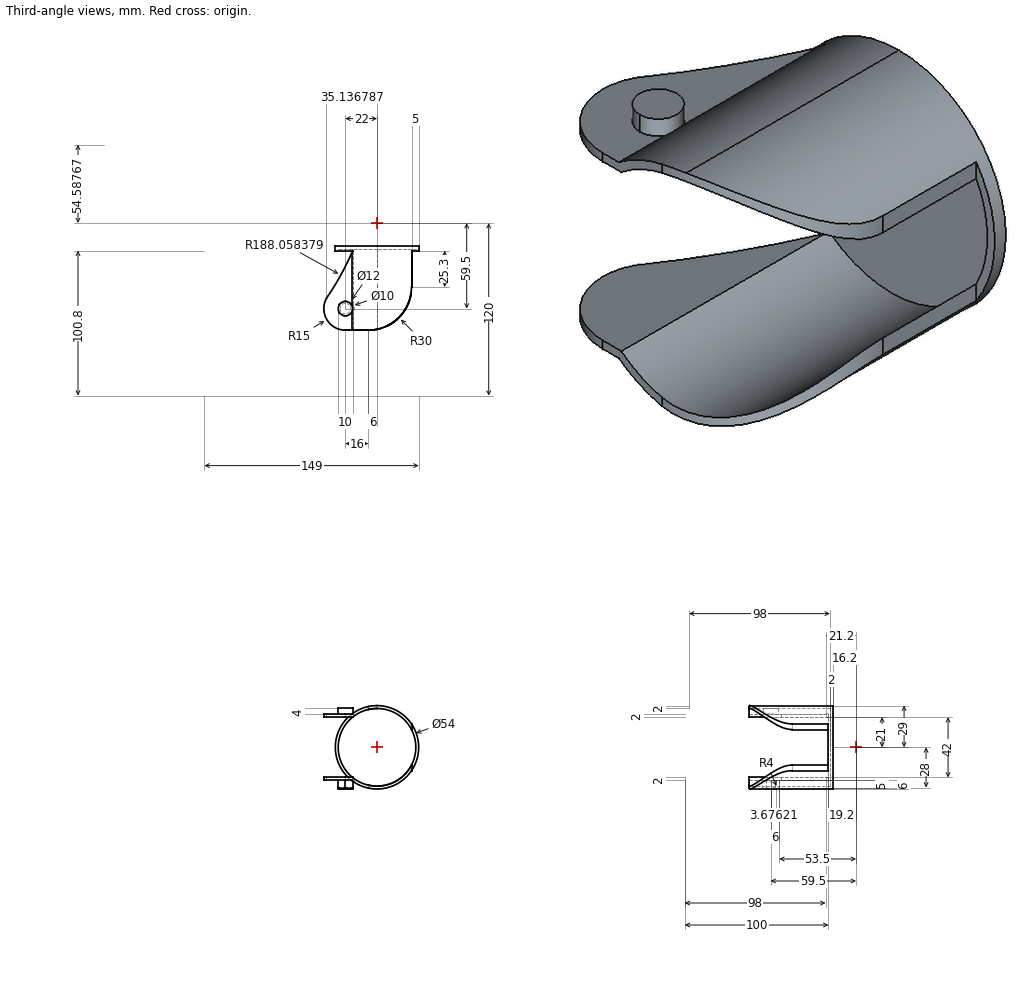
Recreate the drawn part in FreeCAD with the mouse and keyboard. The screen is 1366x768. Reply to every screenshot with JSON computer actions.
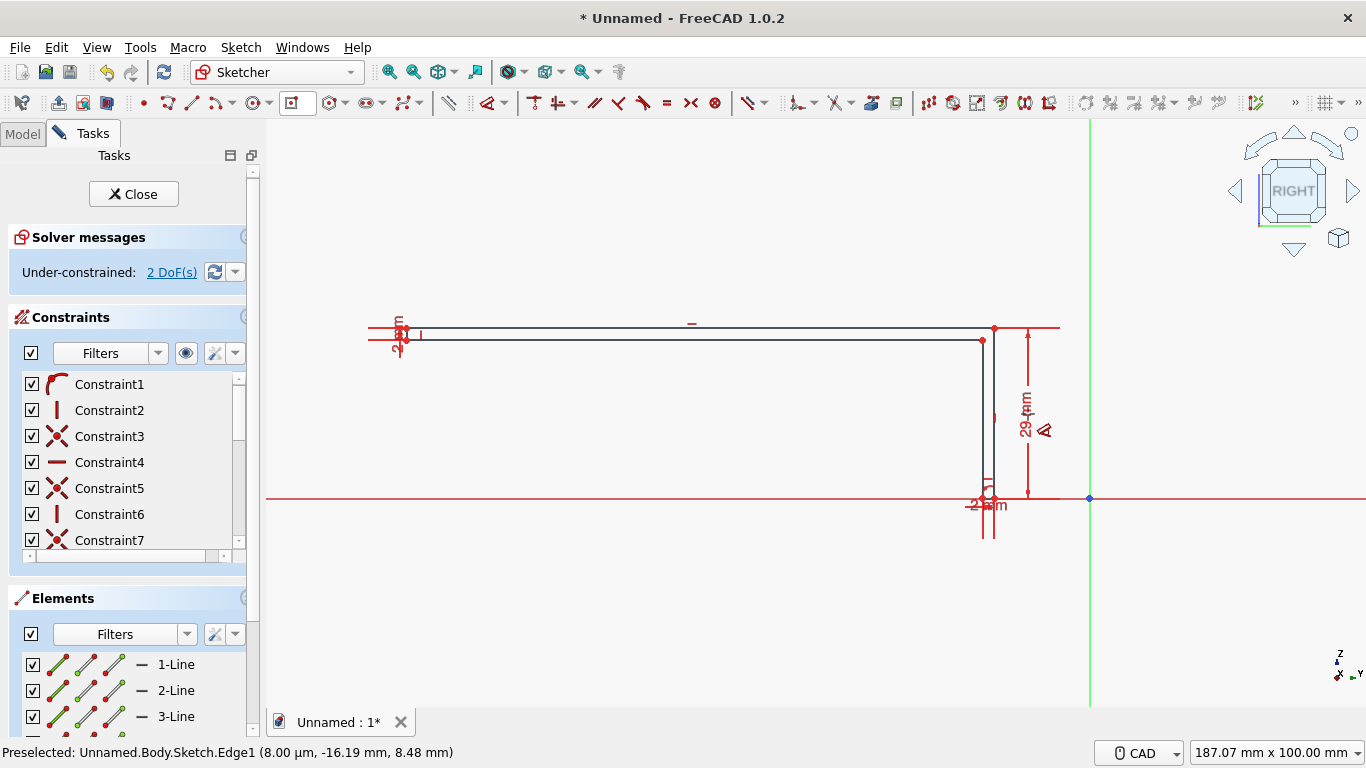
{"action": "left_click", "coordinate": [580, 340]}
{"action": "left_click", "coordinate": [695, 306]}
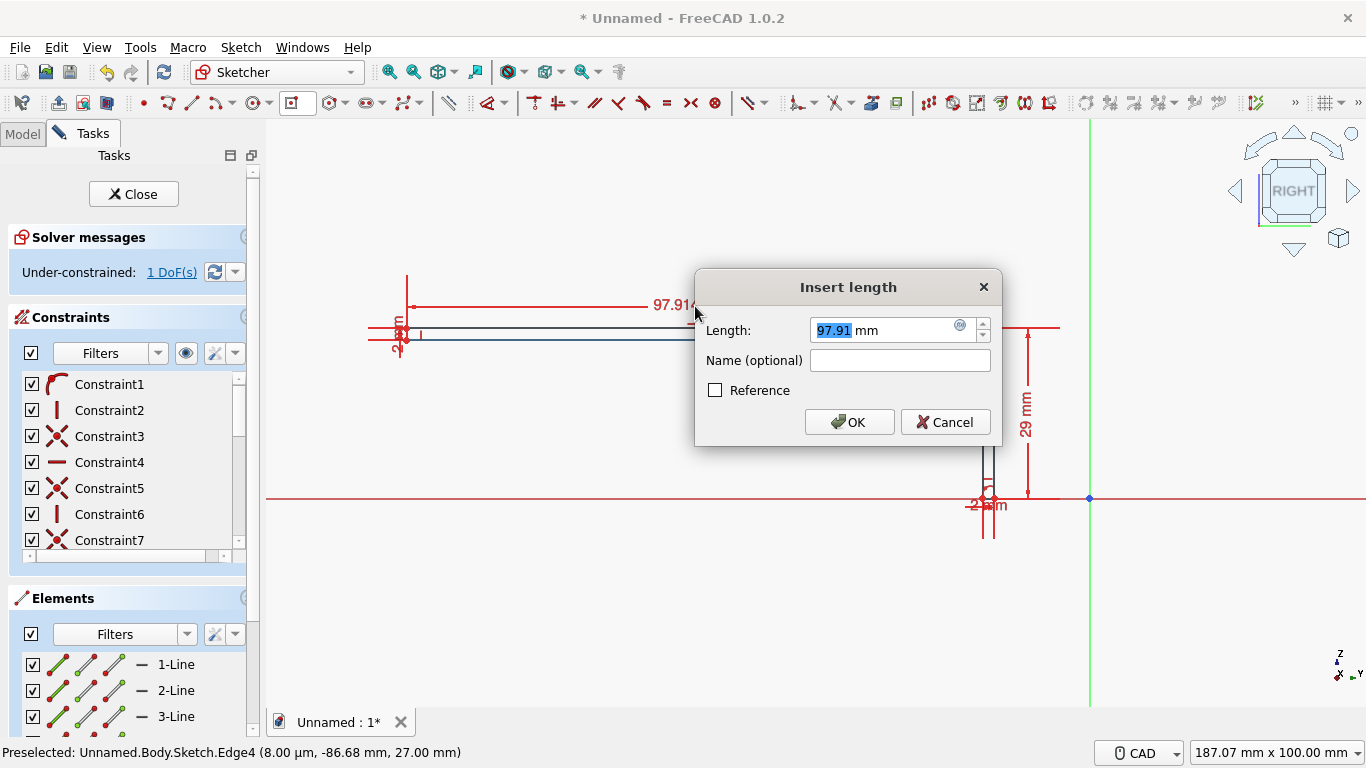
{"action": "type", "text": "98"}
{"action": "key", "text": "Return"}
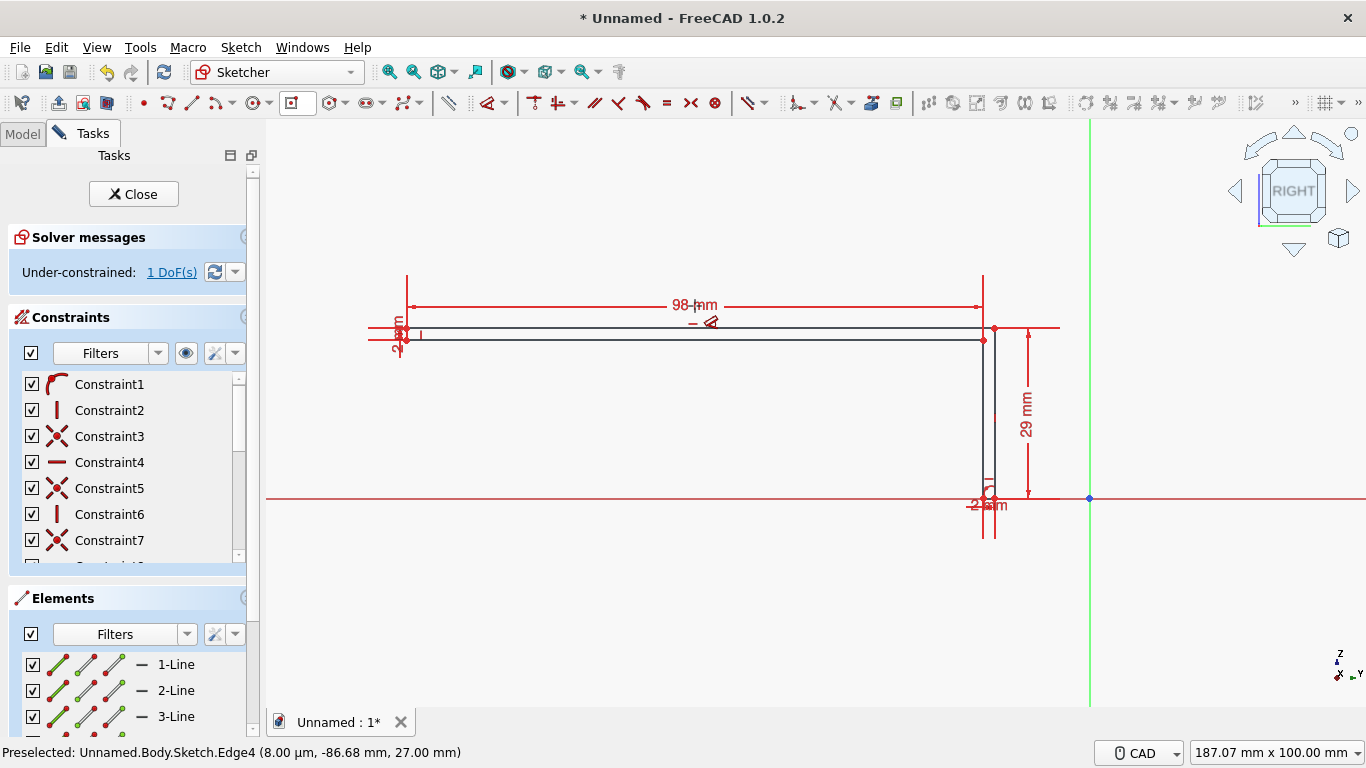
{"action": "left_click", "coordinate": [995, 499]}
{"action": "left_click", "coordinate": [1042, 533]}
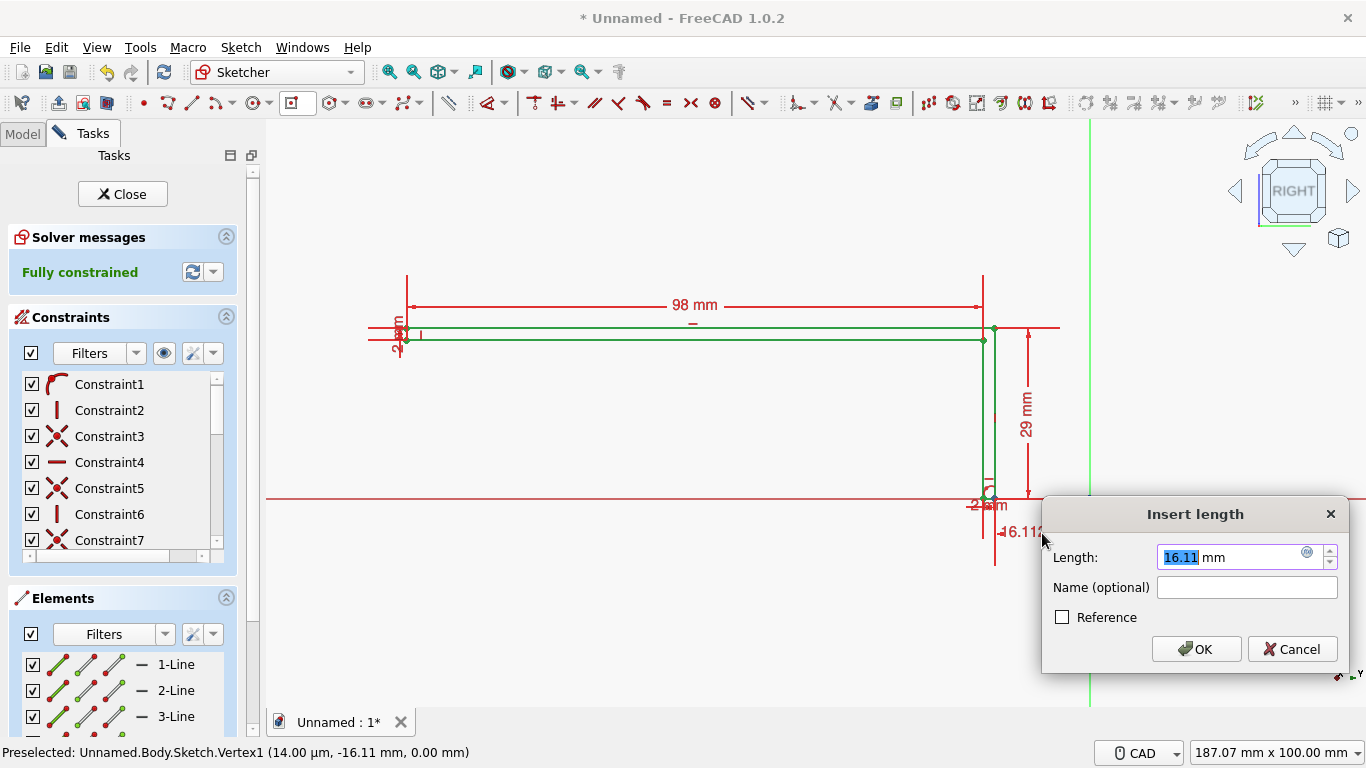
{"action": "type", "text": "16.2"}
{"action": "key", "text": "Return"}
{"action": "key", "text": "Escape"}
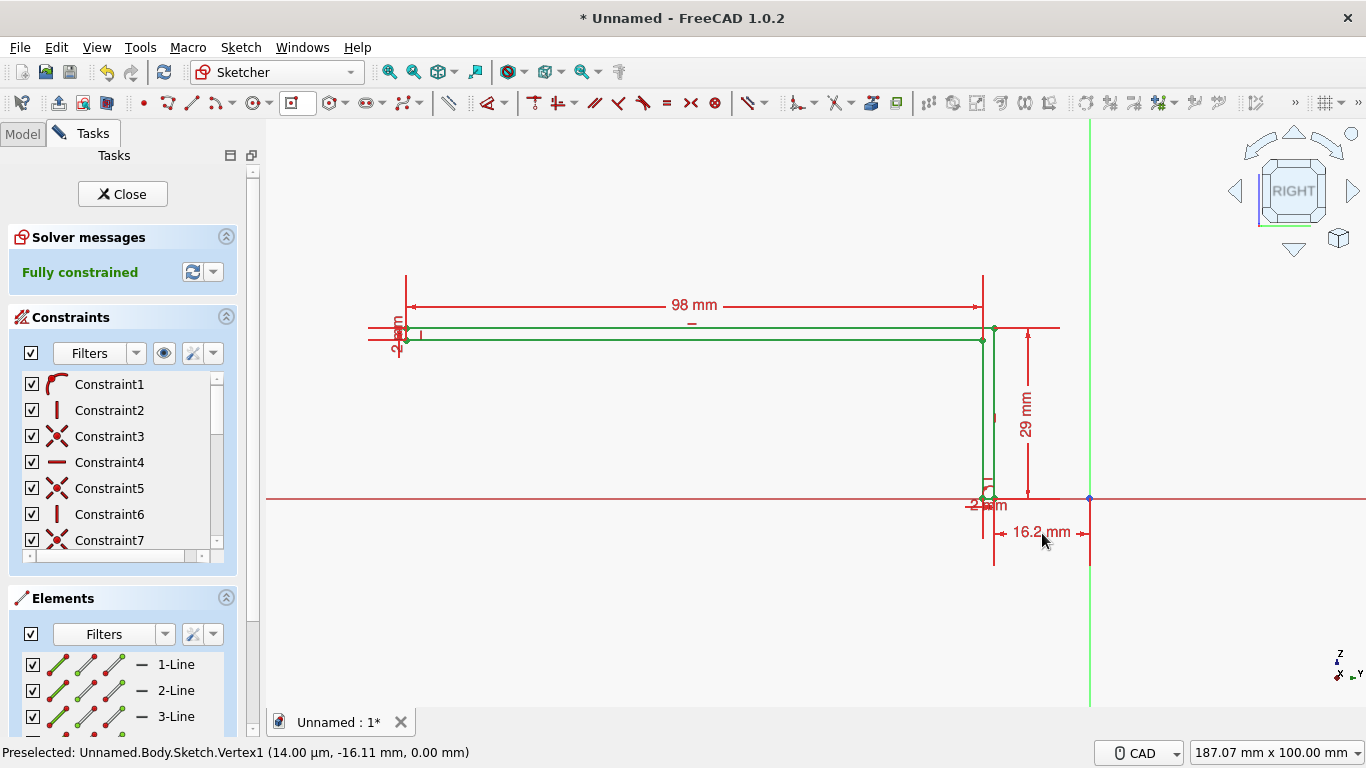
{"action": "left_click", "coordinate": [123, 194]}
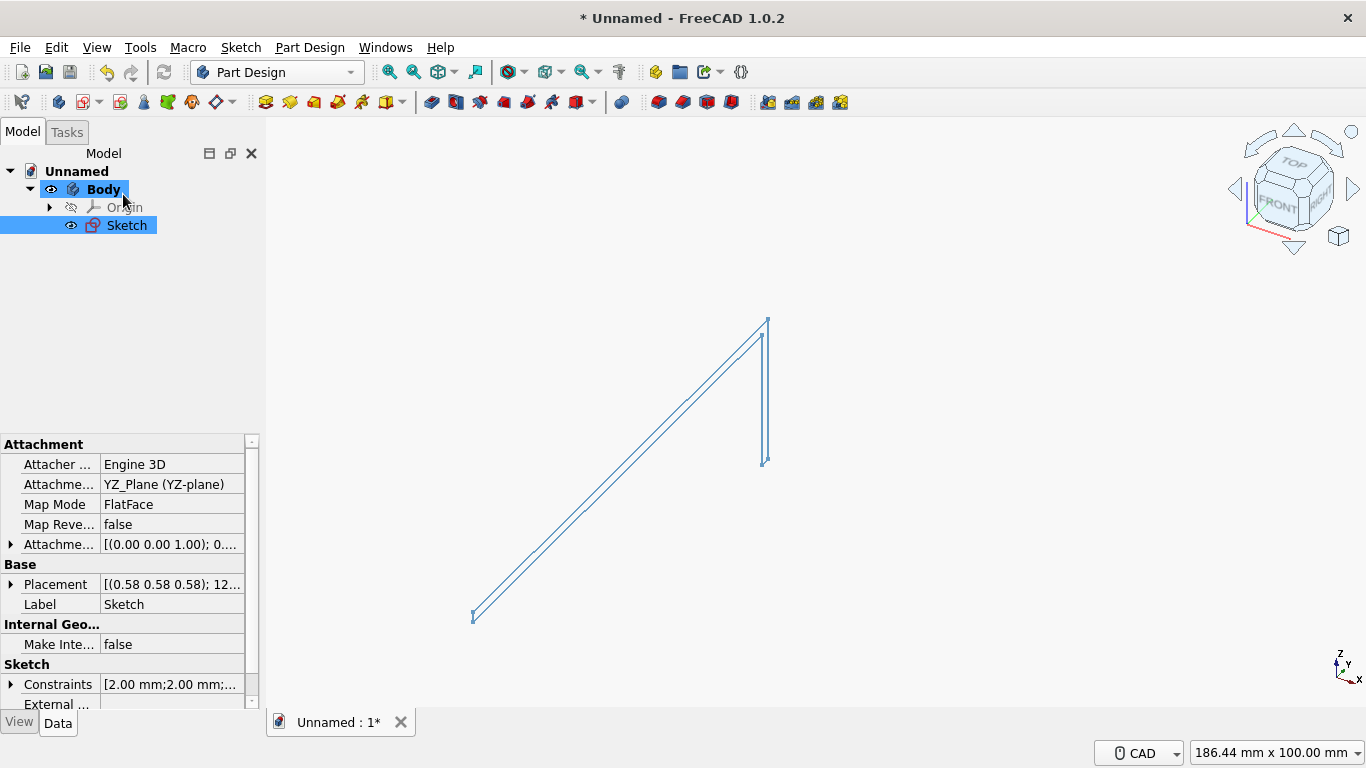
{"action": "left_click", "coordinate": [290, 102]}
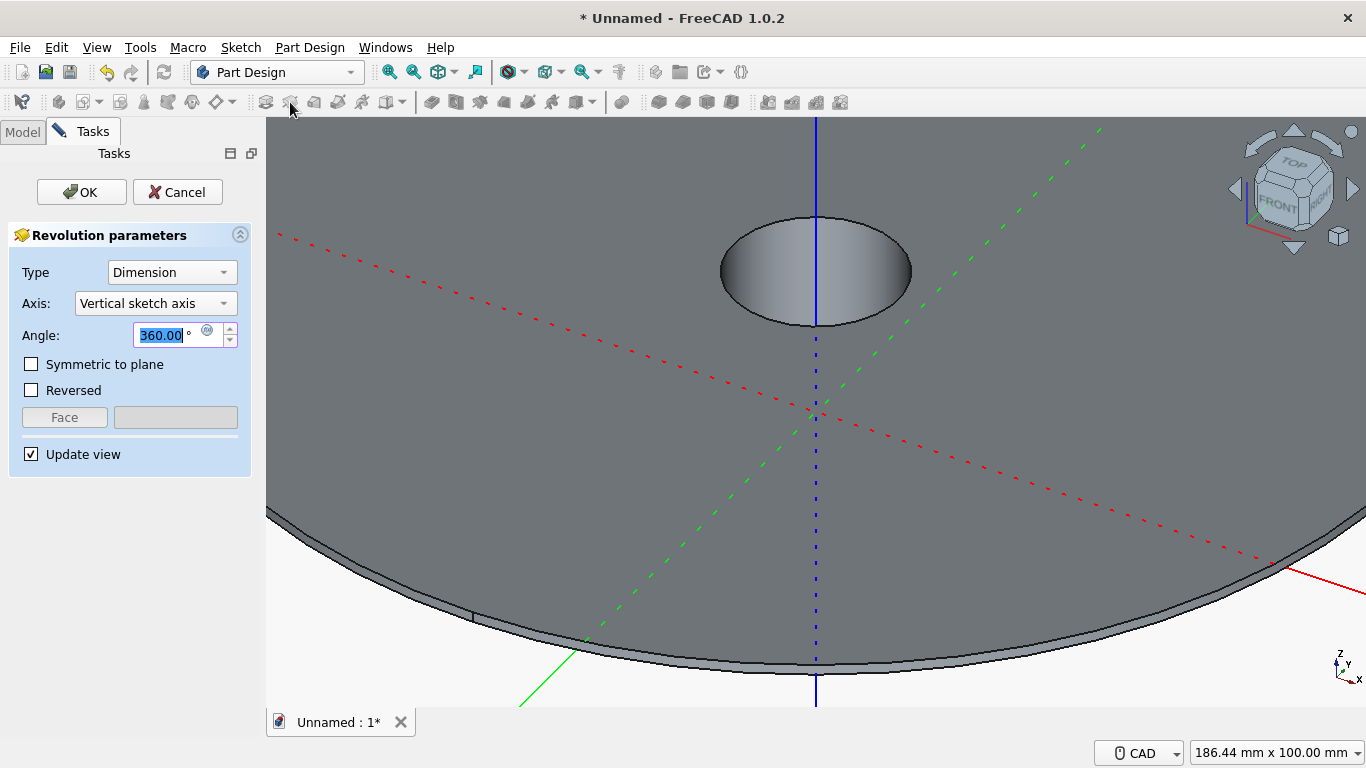
{"action": "left_click", "coordinate": [156, 304]}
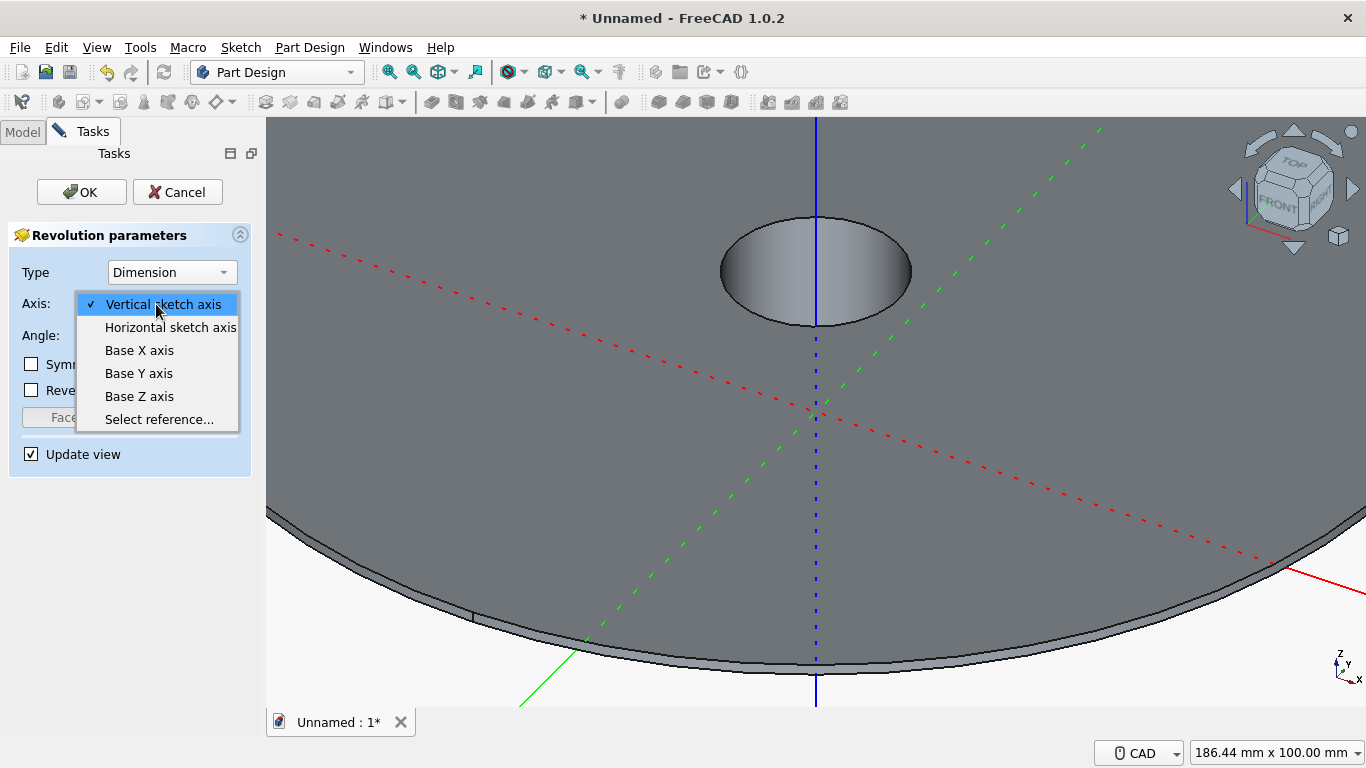
{"action": "left_click", "coordinate": [156, 328]}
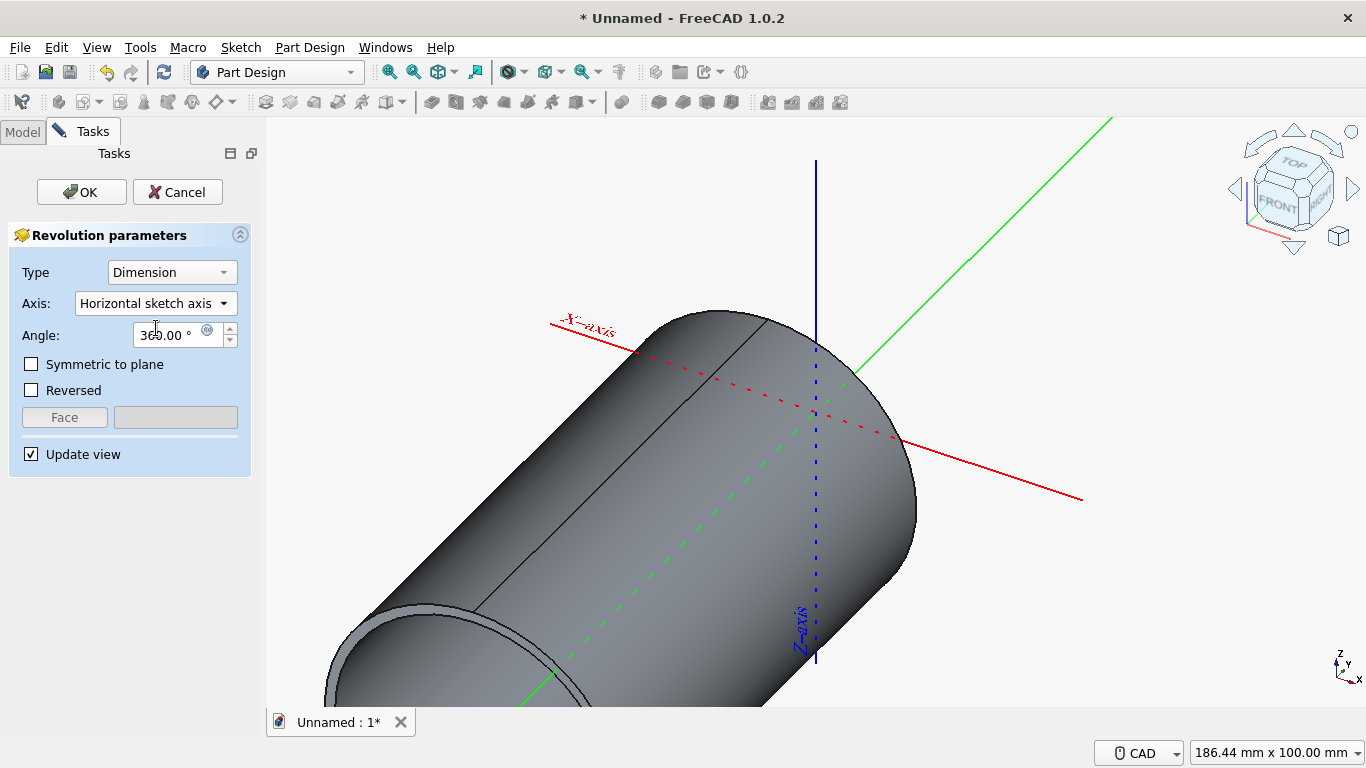
{"action": "left_click", "coordinate": [82, 192]}